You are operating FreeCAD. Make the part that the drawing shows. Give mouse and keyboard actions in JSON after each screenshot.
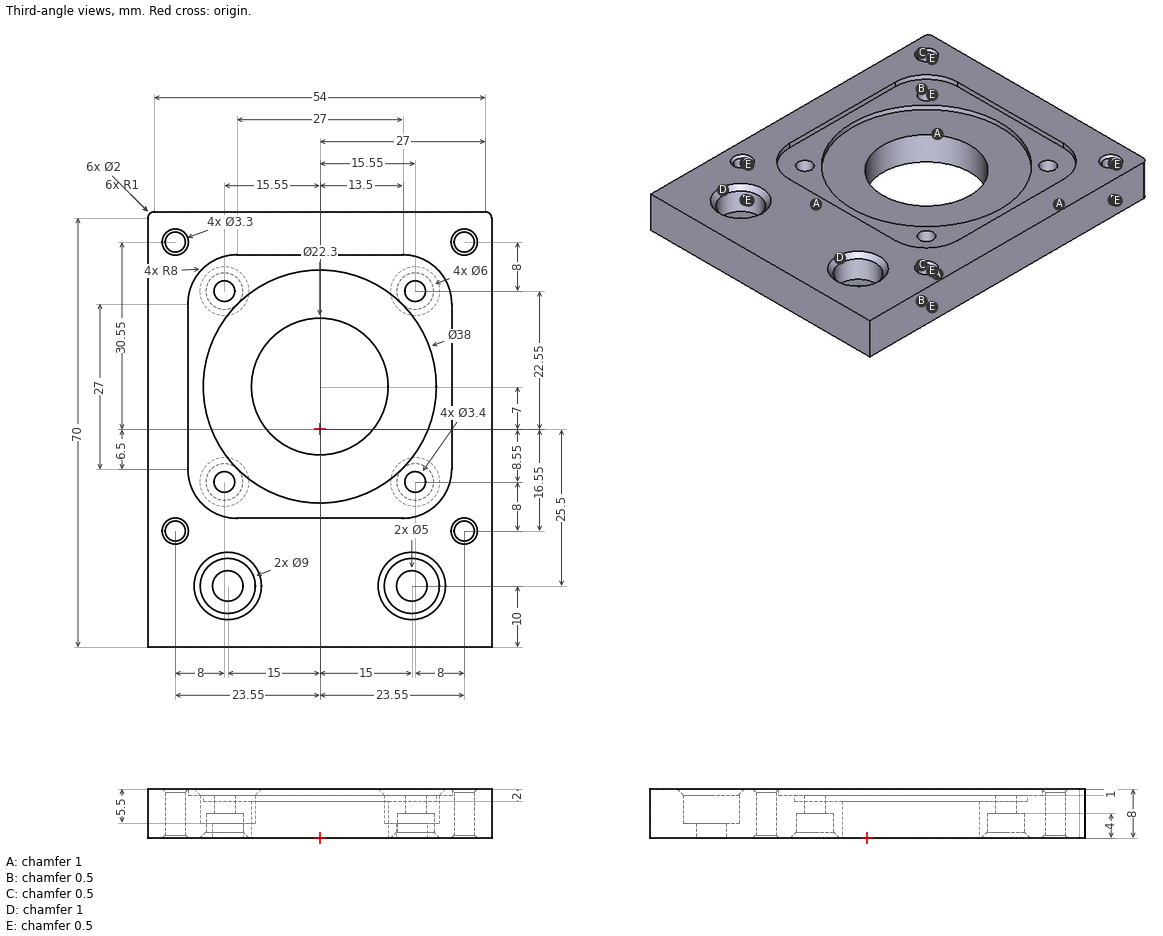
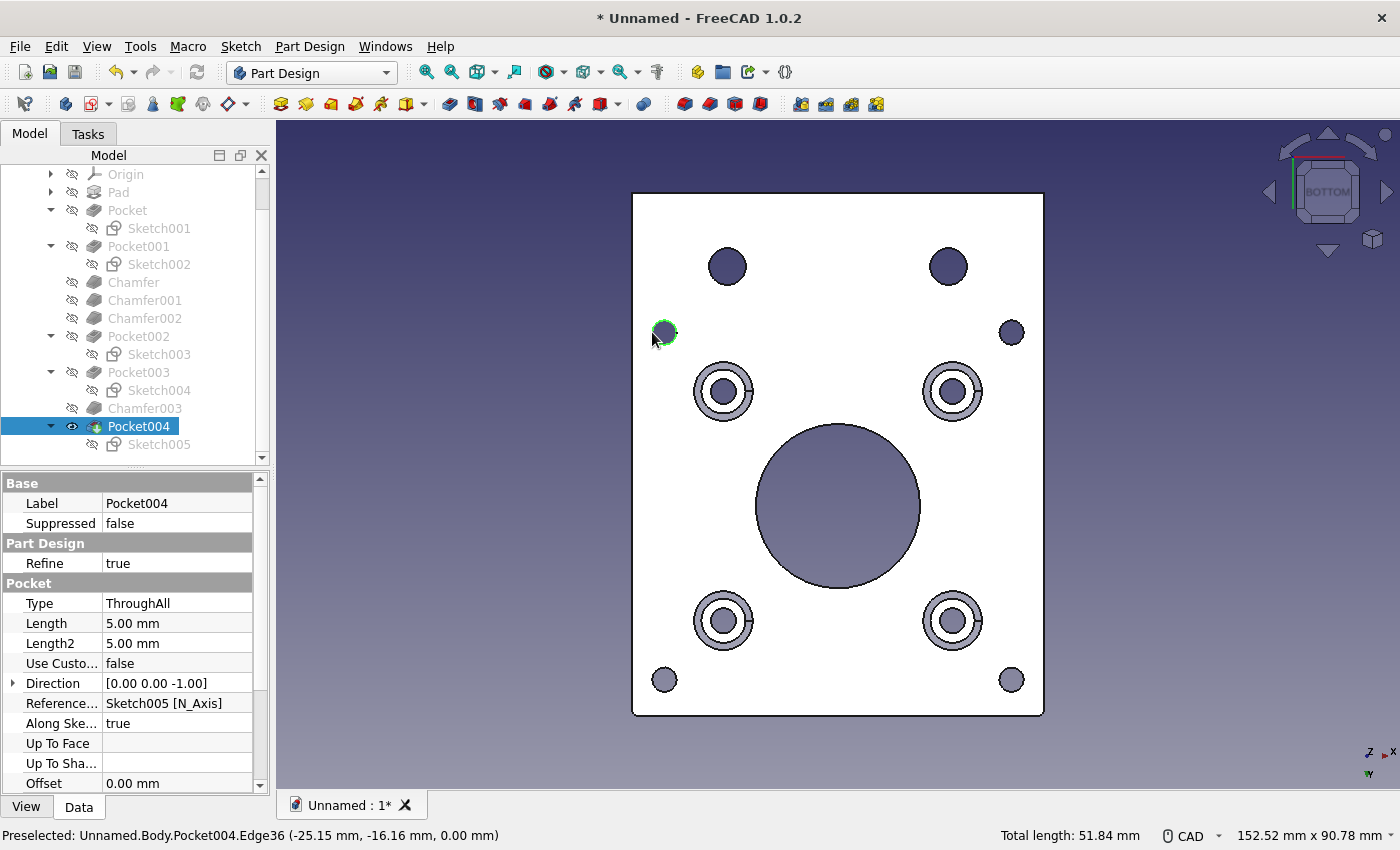
{"action": "left_click", "coordinate": [1002, 339], "text": "ctrl"}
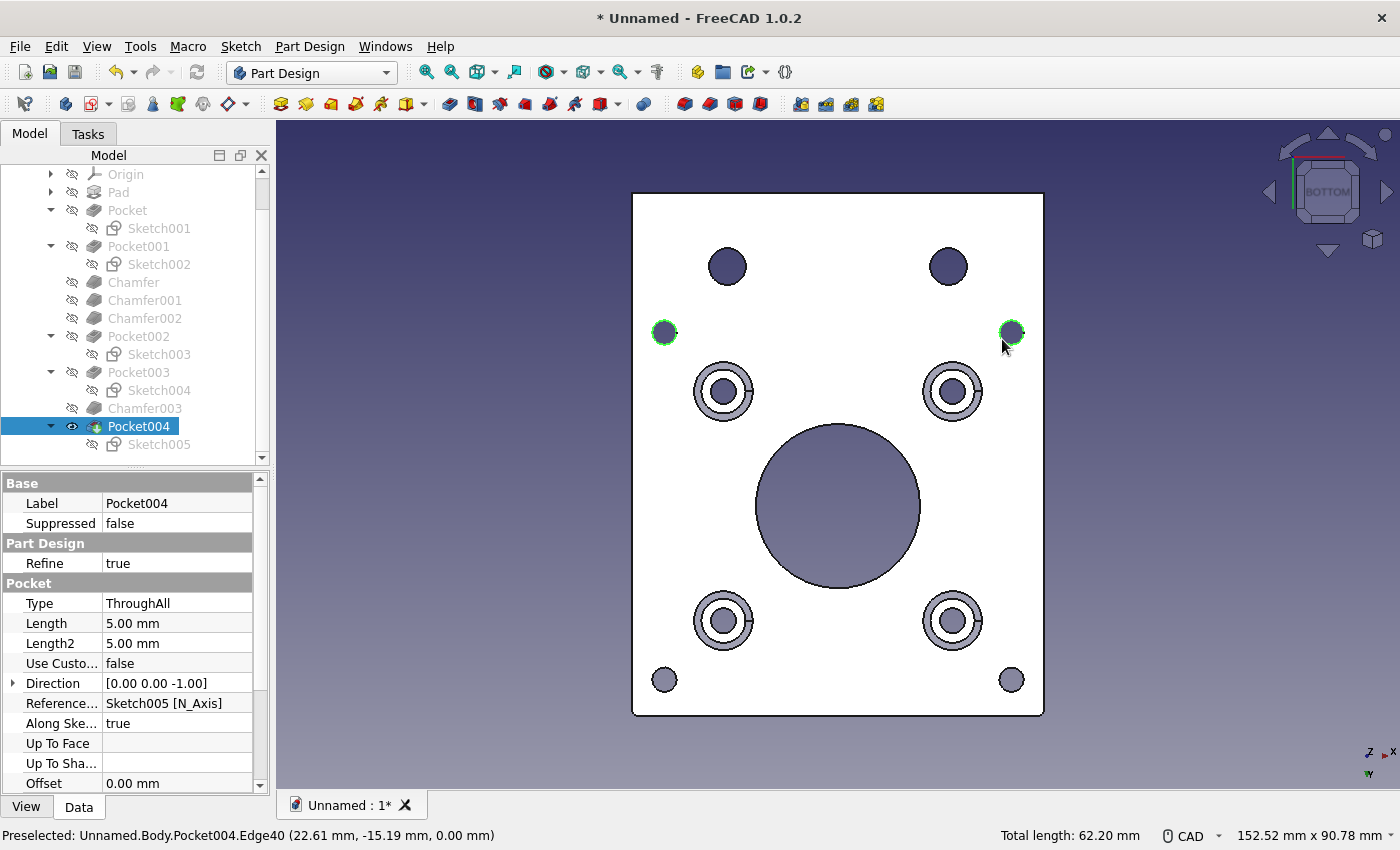
{"action": "left_click", "coordinate": [999, 679], "text": "ctrl"}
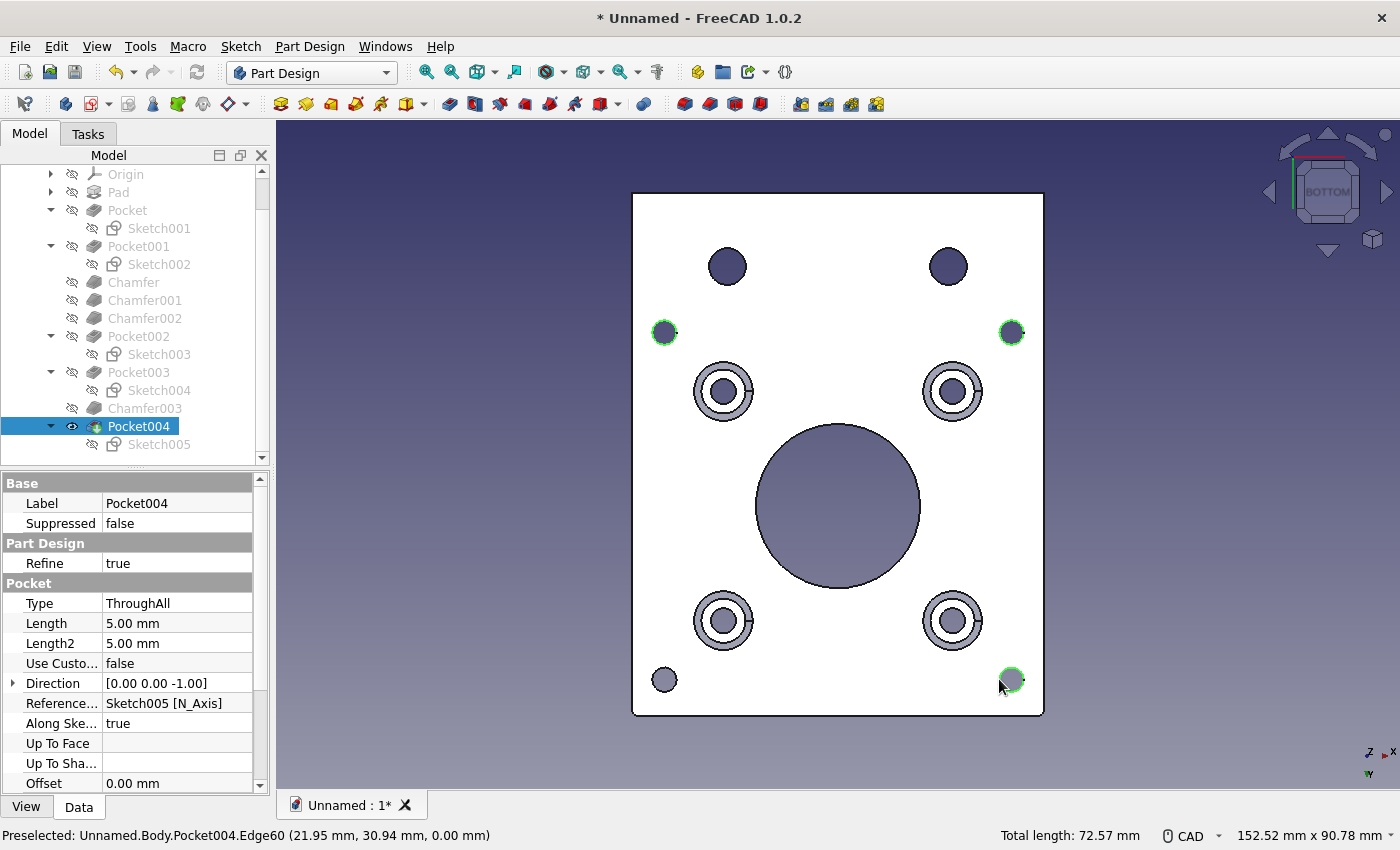
{"action": "left_click", "coordinate": [652, 679], "text": "ctrl"}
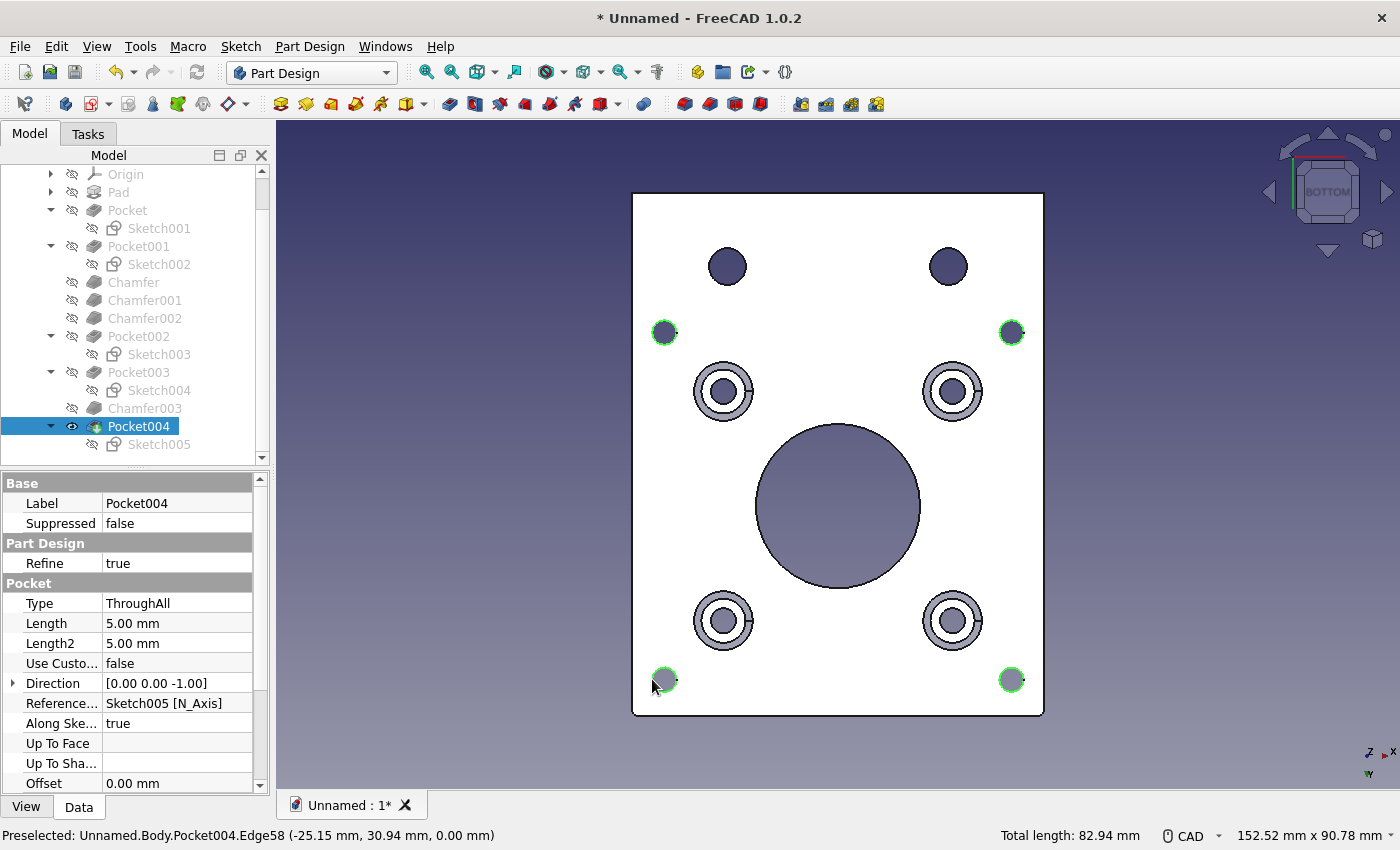
{"action": "left_click", "coordinate": [710, 104]}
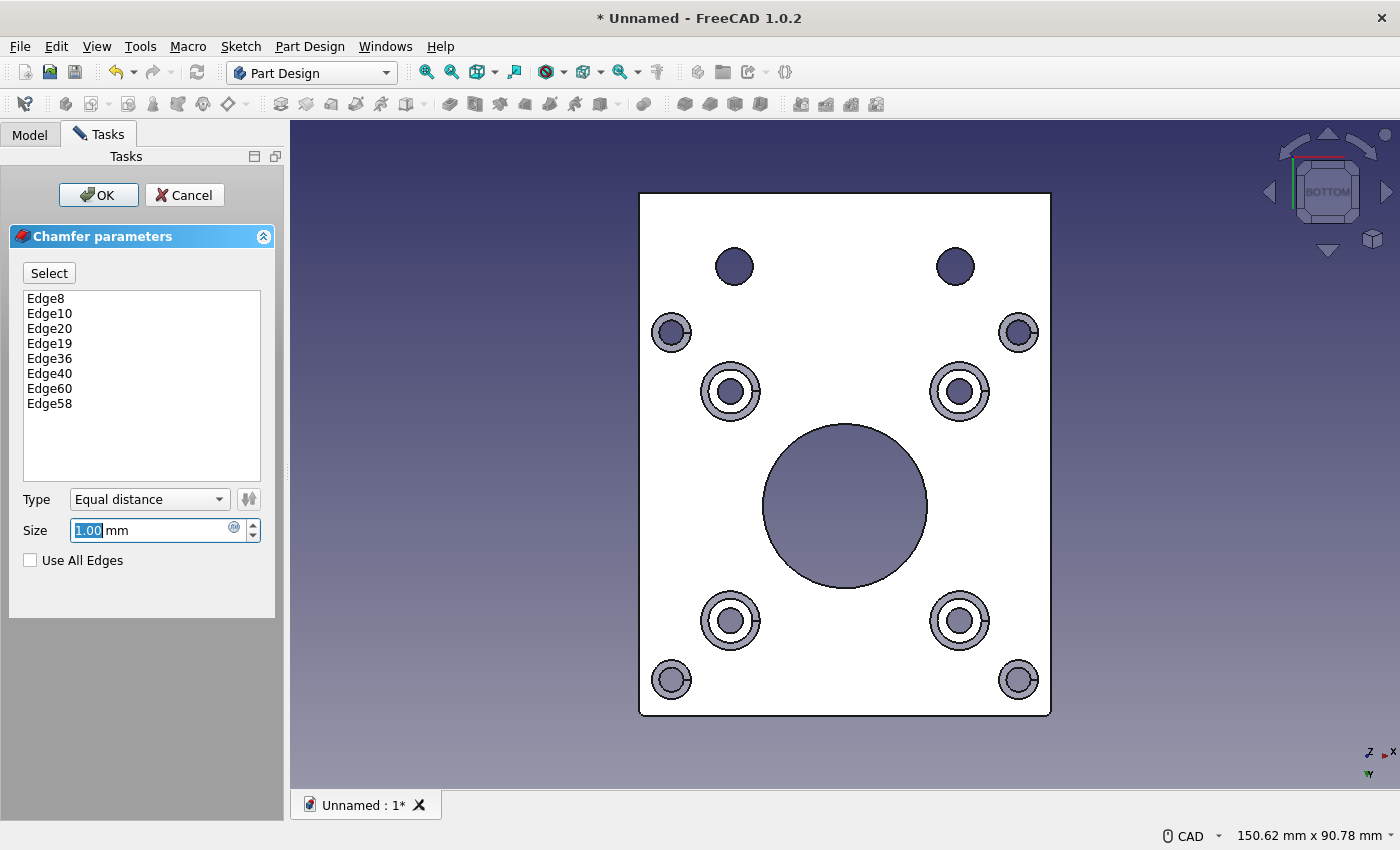
{"action": "type", "text": "0.5"}
{"action": "key", "text": "Tab"}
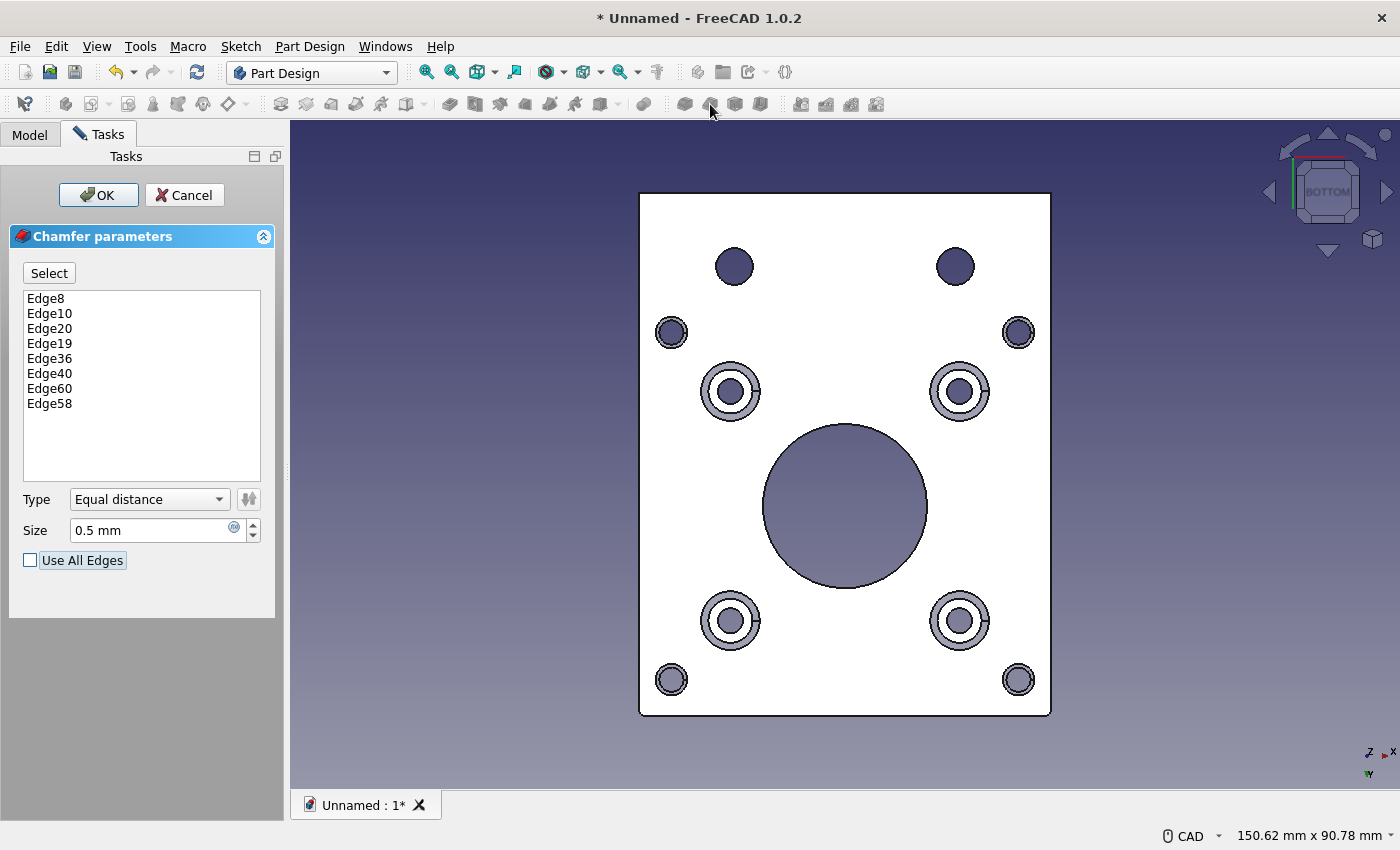
{"action": "left_click", "coordinate": [99, 195]}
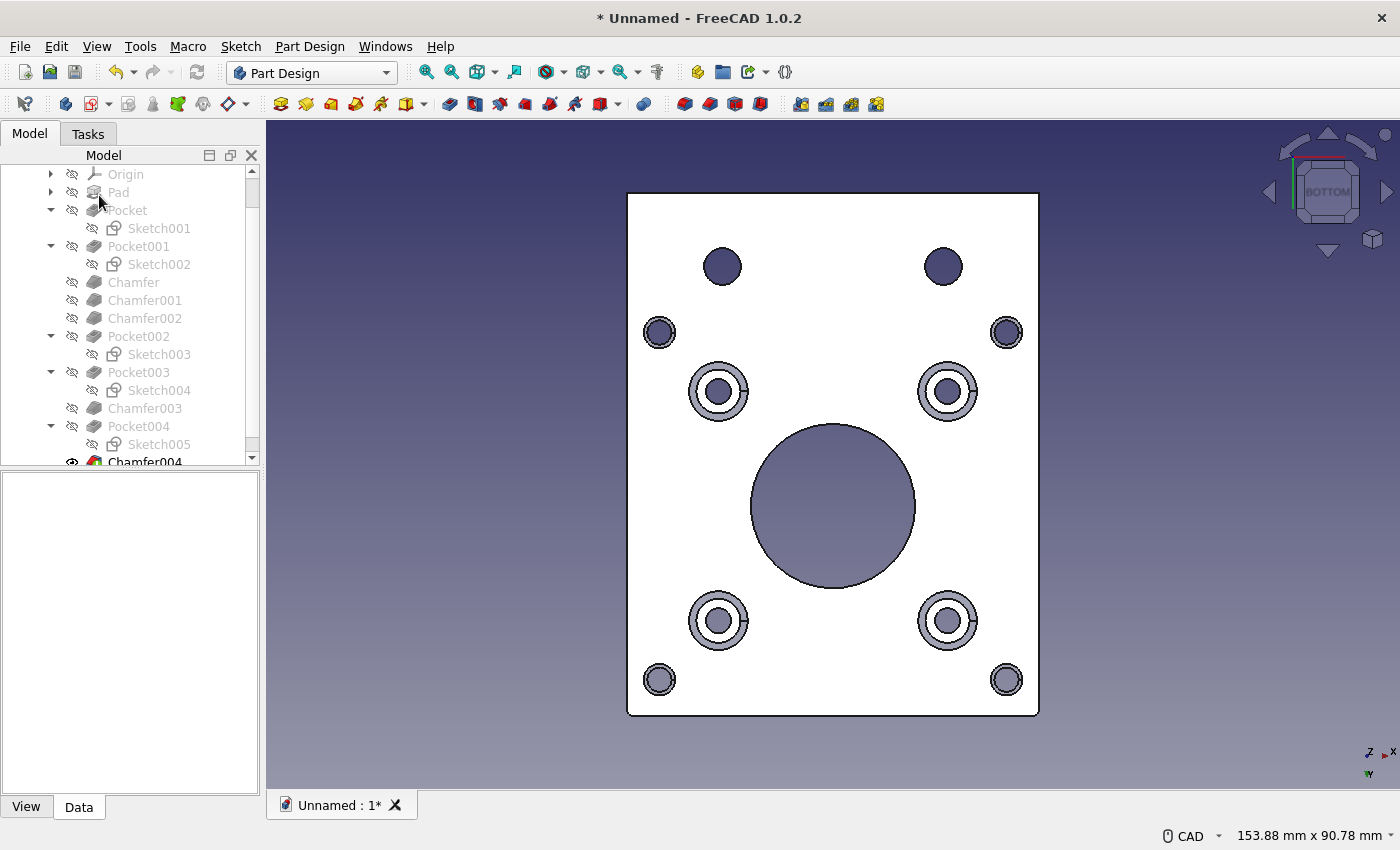
{"action": "key", "text": "0"}